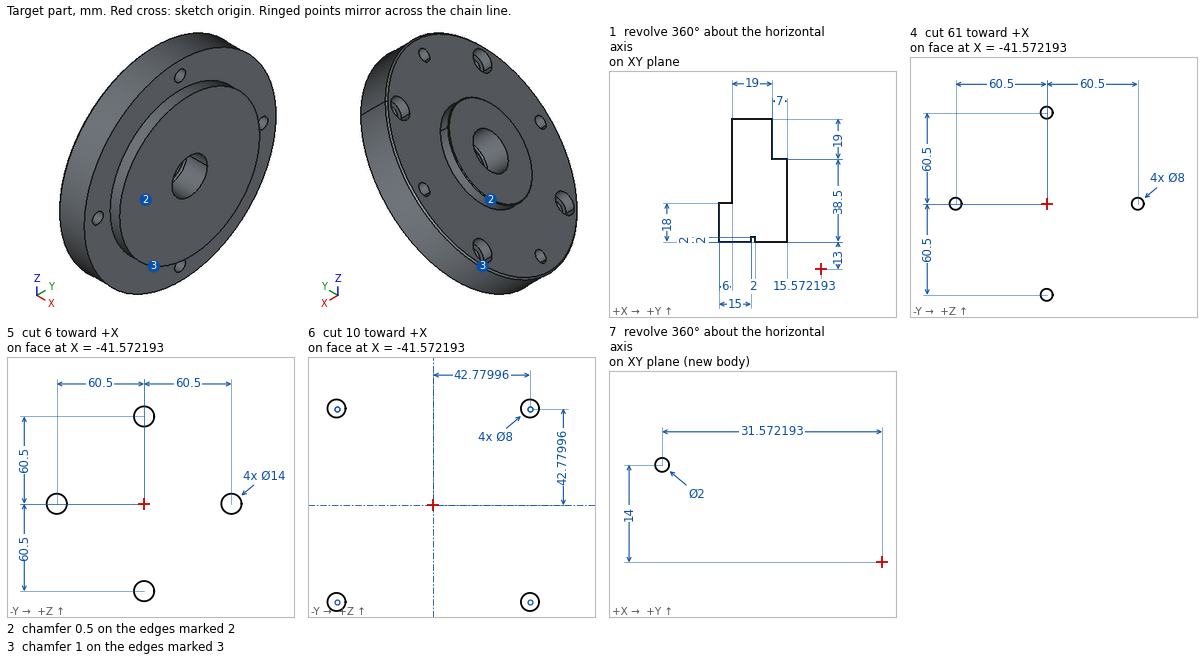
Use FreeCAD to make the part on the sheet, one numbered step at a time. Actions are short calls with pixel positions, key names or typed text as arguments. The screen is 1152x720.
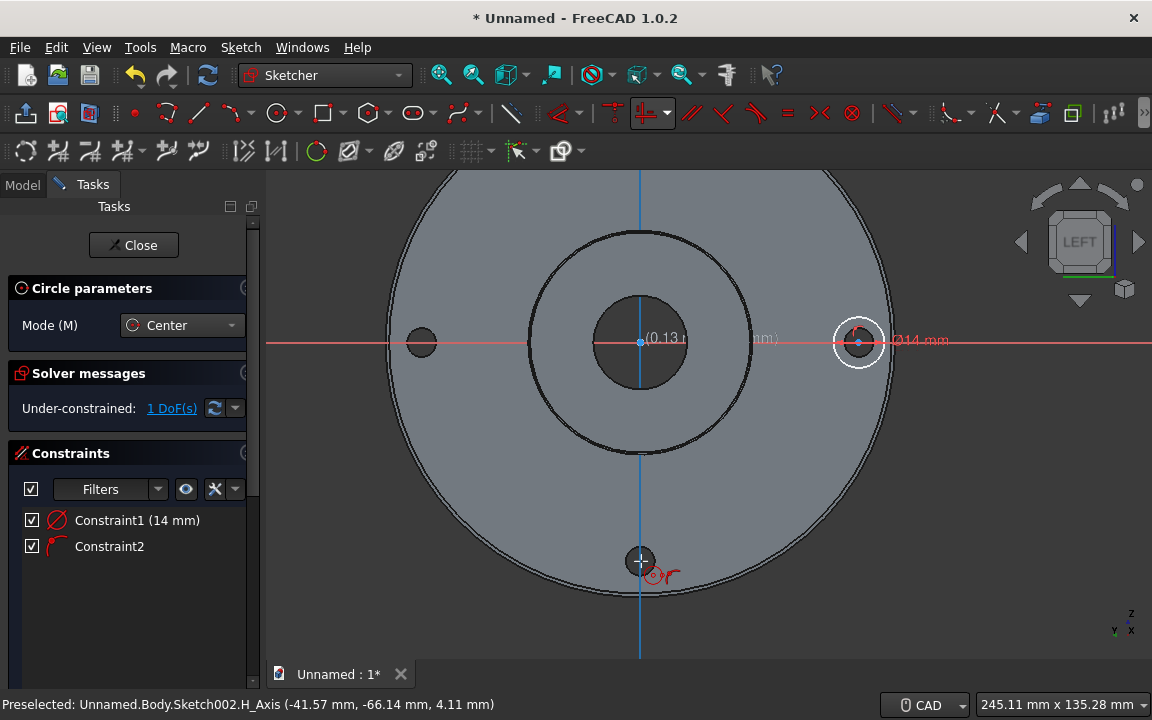
click(640, 561)
move(658, 543)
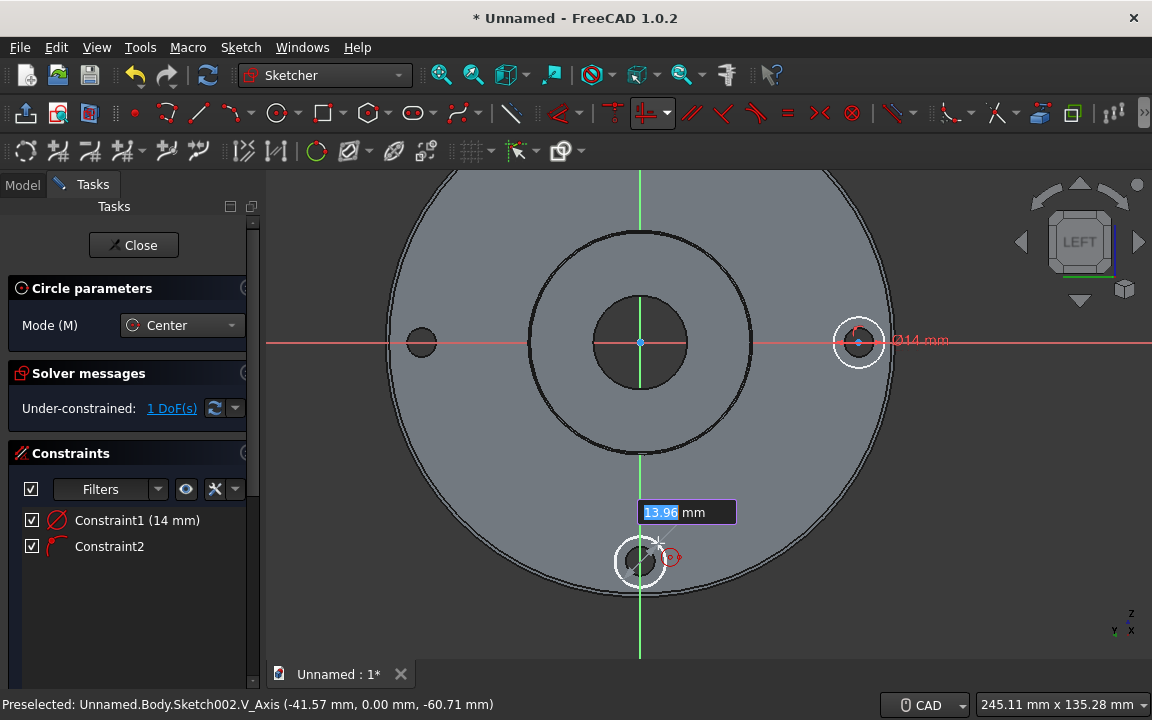
text(14)
key(Return)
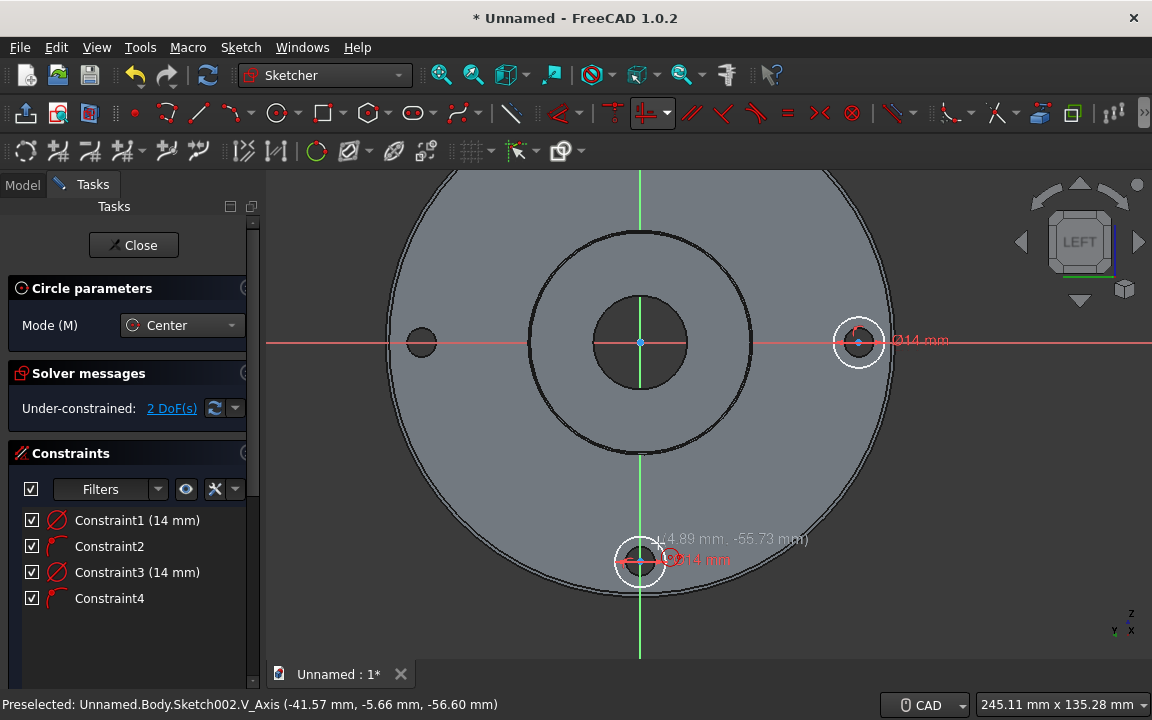
scroll(641, 561, down, 2)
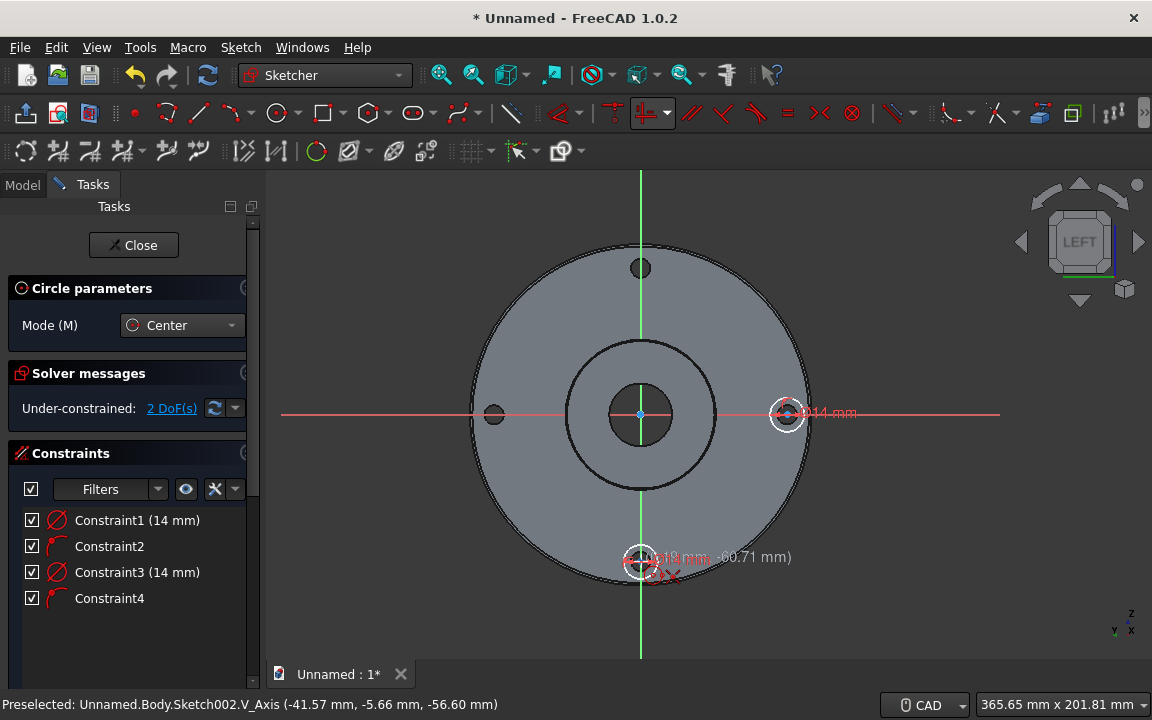
scroll(641, 268, up, 2)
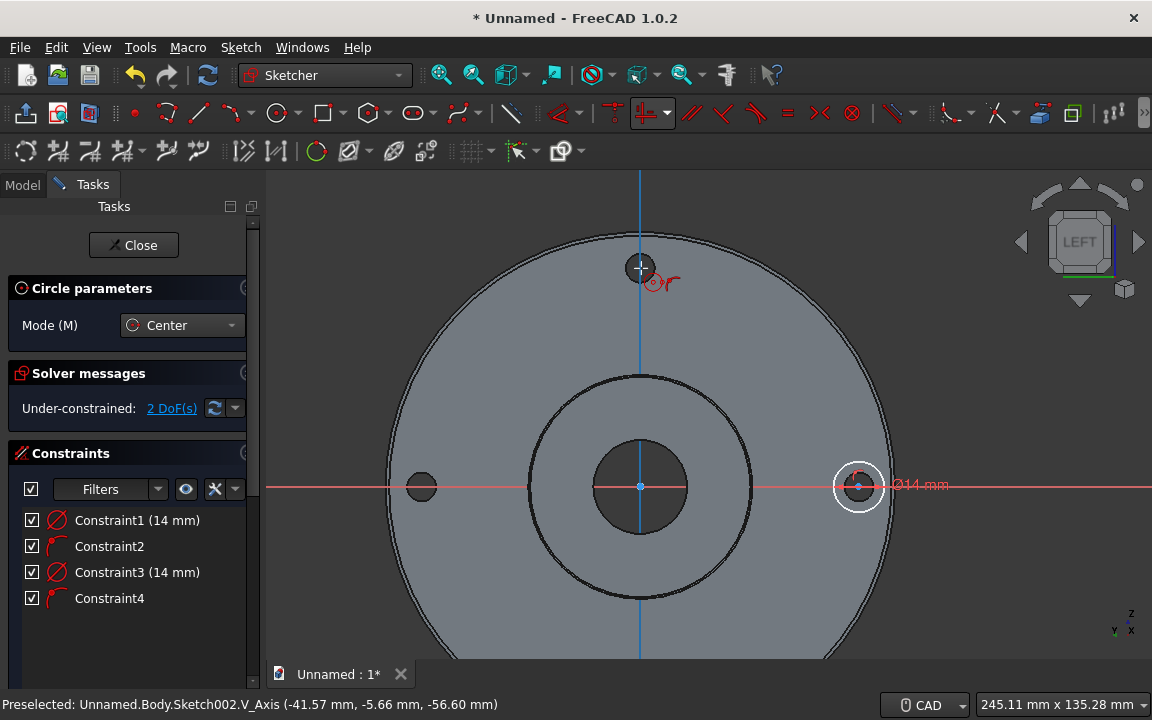
click(640, 268)
move(658, 250)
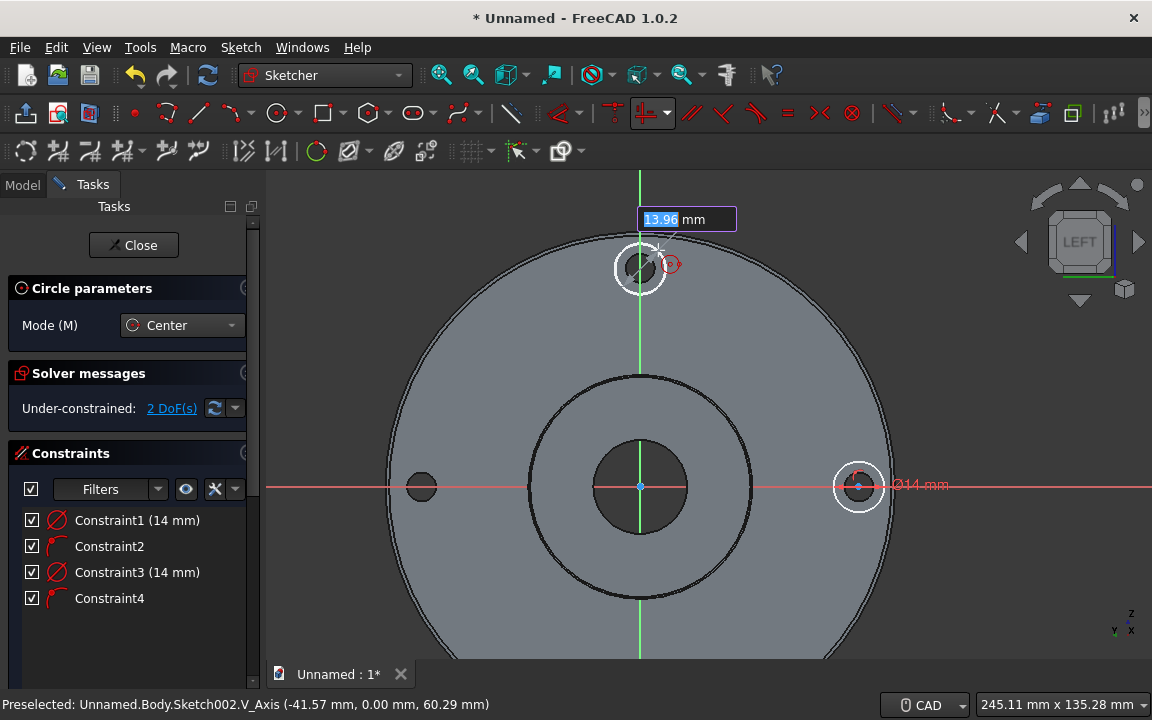
text(14)
key(Return)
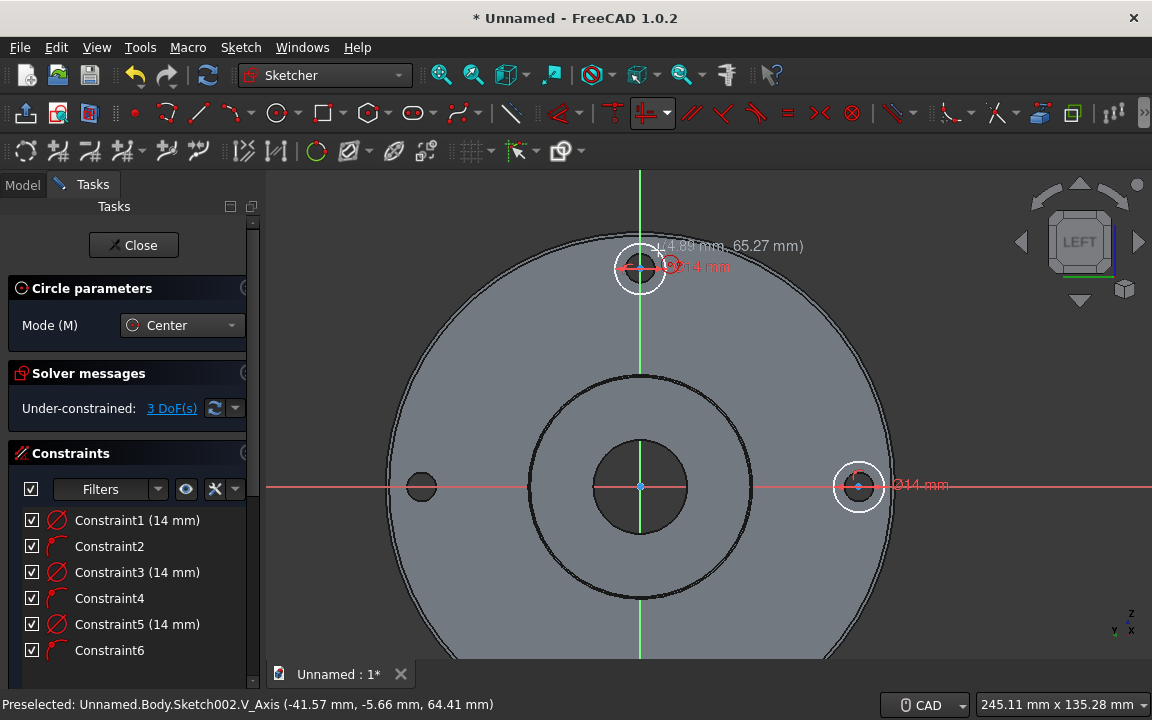
click(422, 487)
move(440, 469)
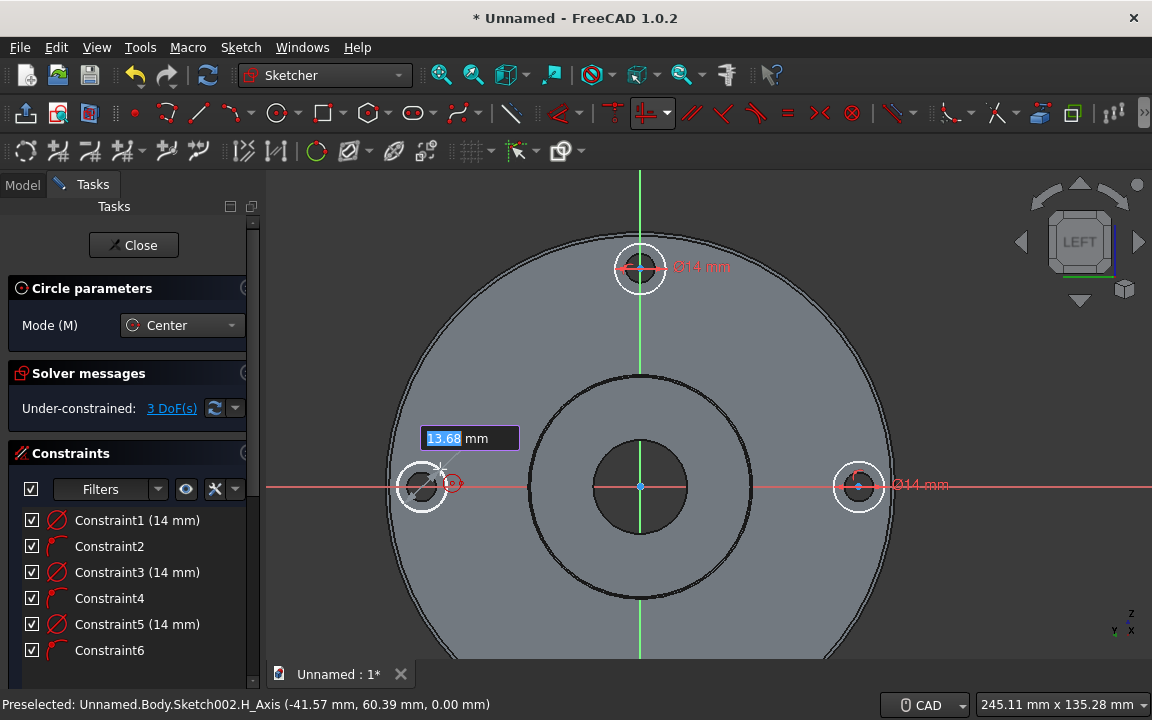
text(14)
key(Return)
key(Escape)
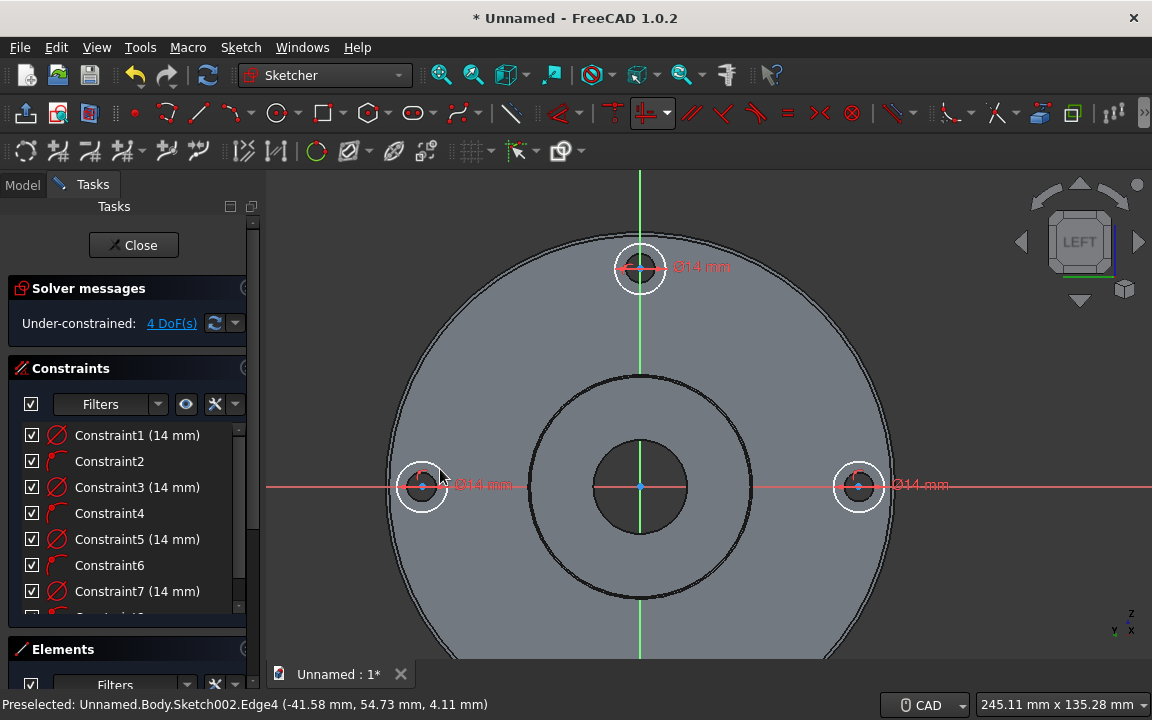
click(558, 114)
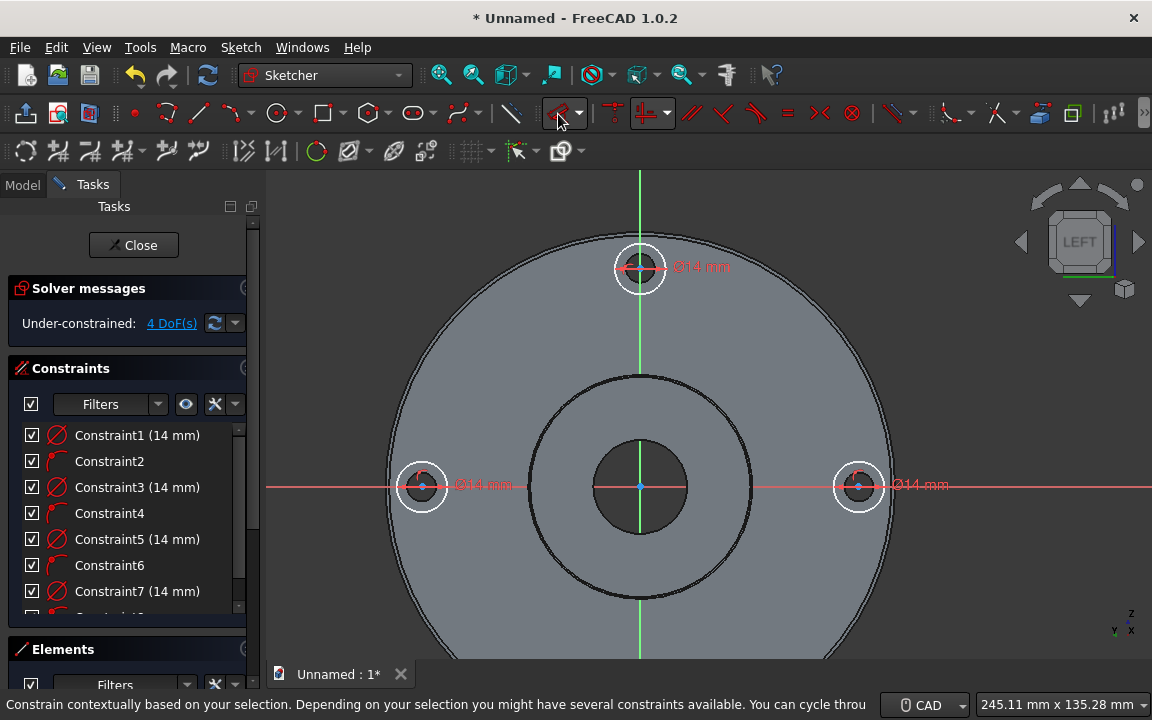
click(859, 487)
click(750, 521)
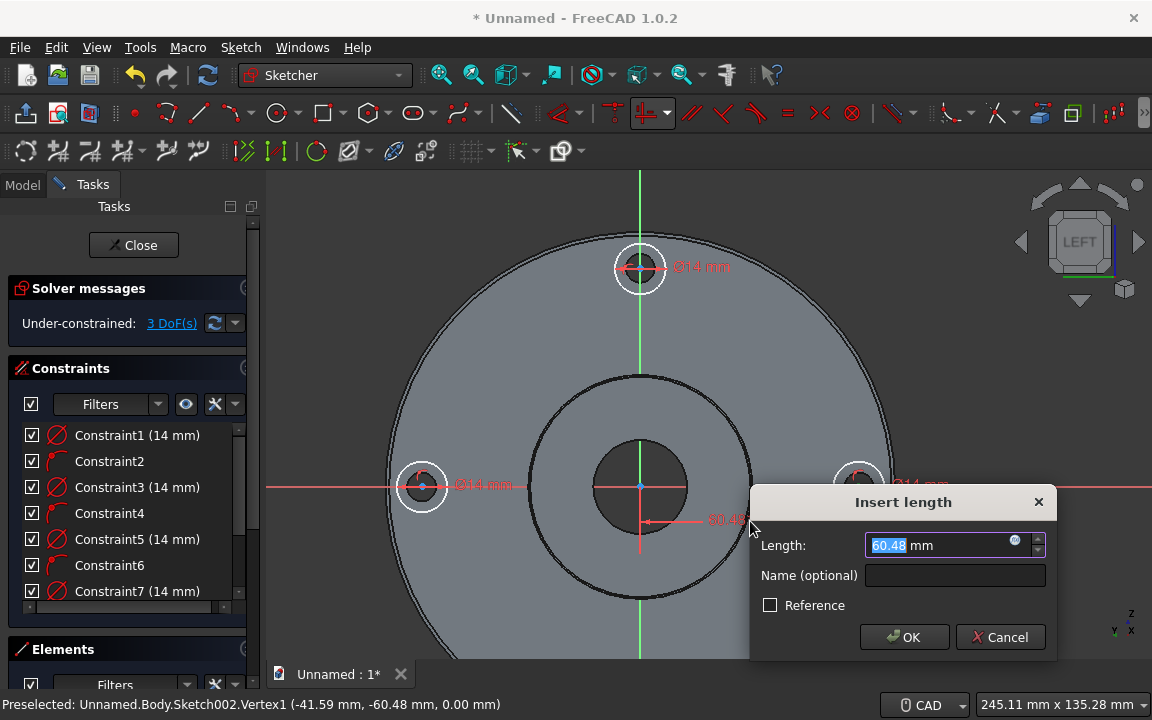
text(60.5)
key(Return)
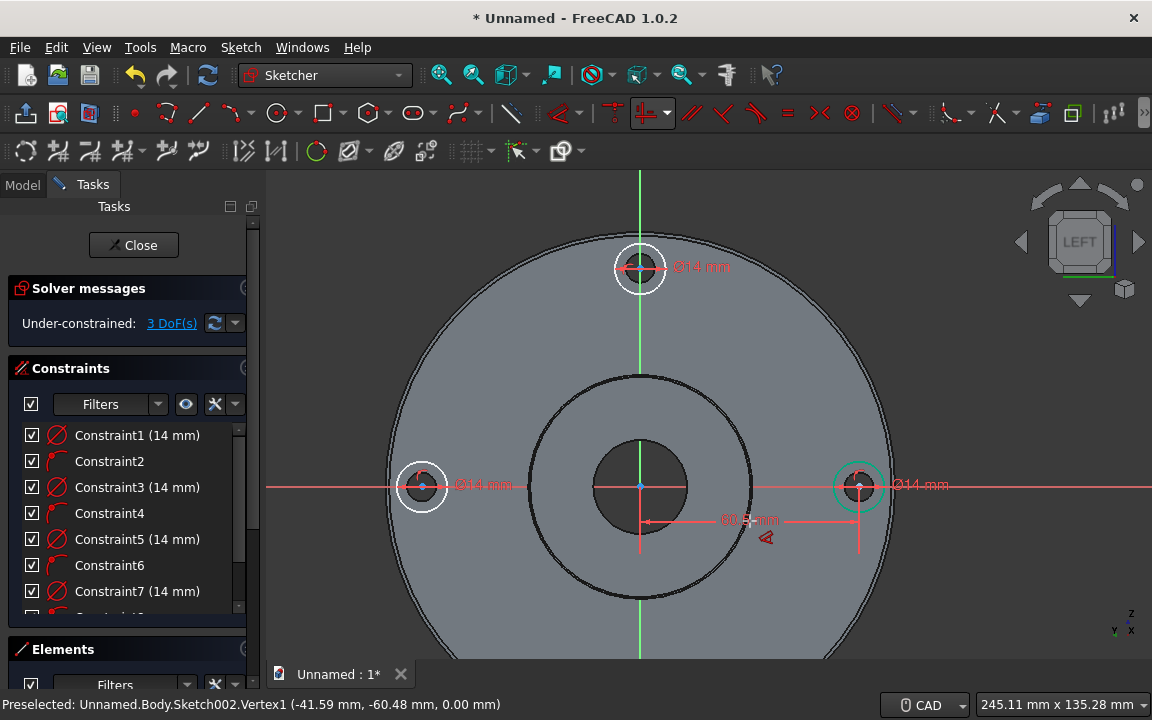
scroll(641, 267, down, 2)